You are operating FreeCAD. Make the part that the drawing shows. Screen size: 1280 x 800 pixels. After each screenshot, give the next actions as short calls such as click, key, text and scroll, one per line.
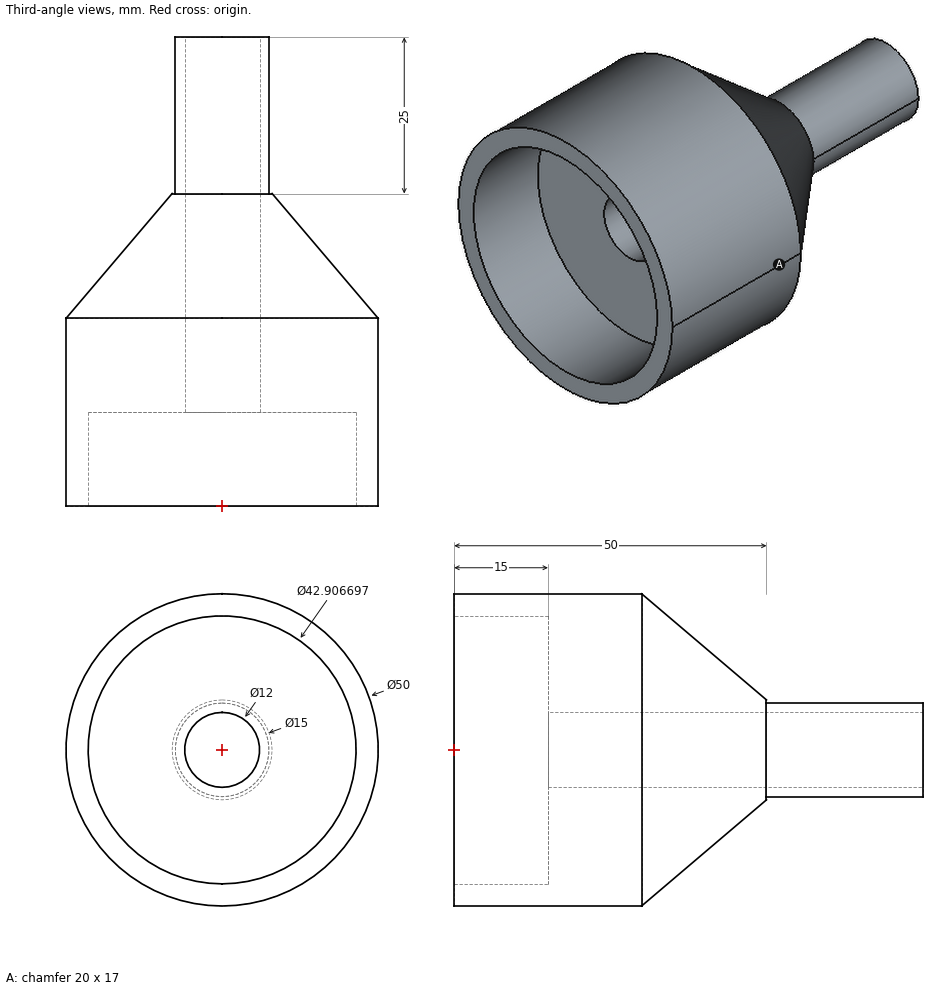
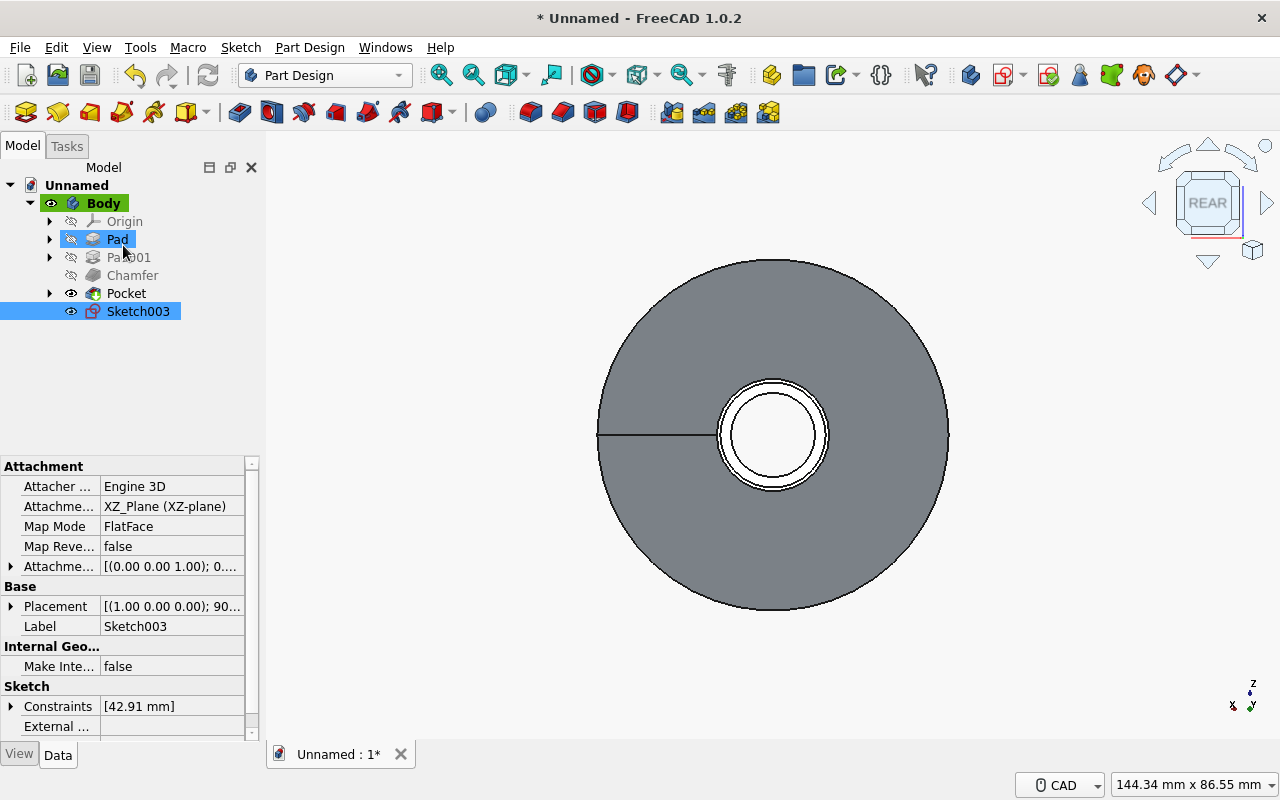
click(240, 112)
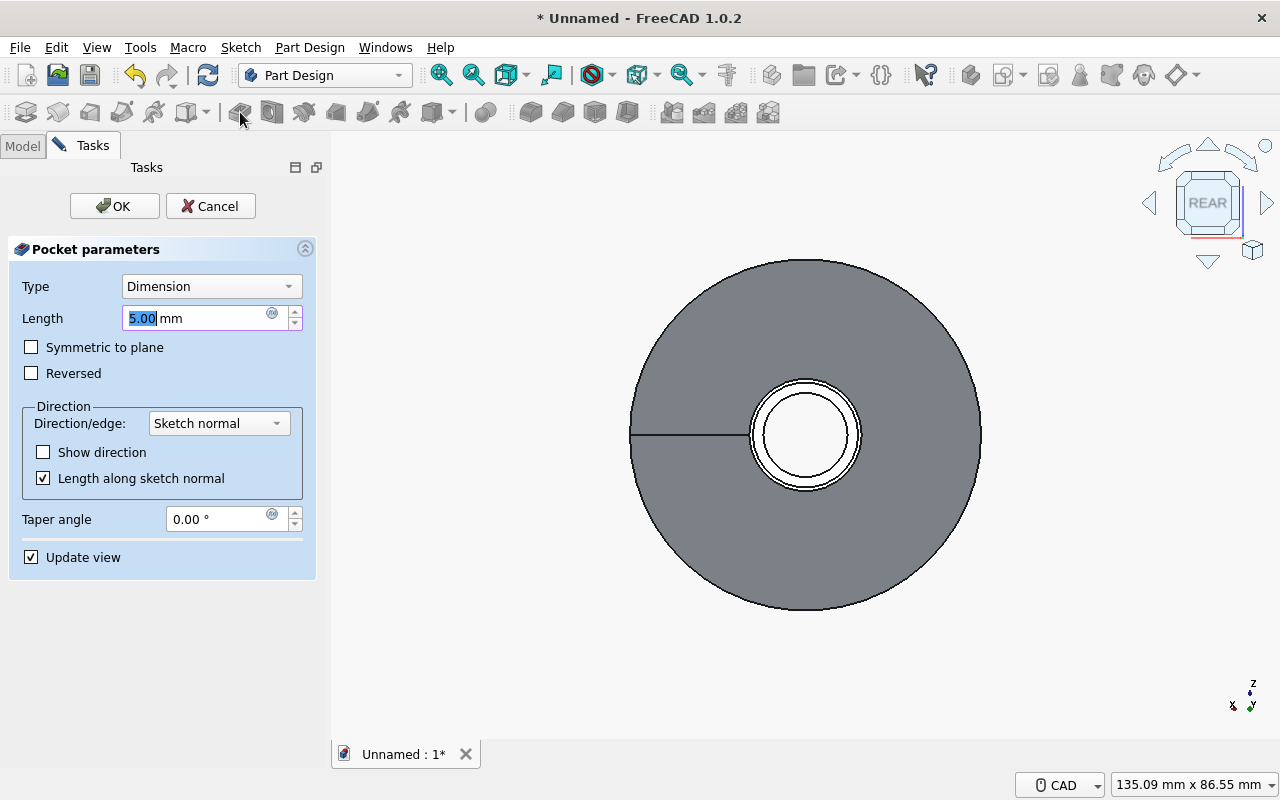
text(15)
key(Tab)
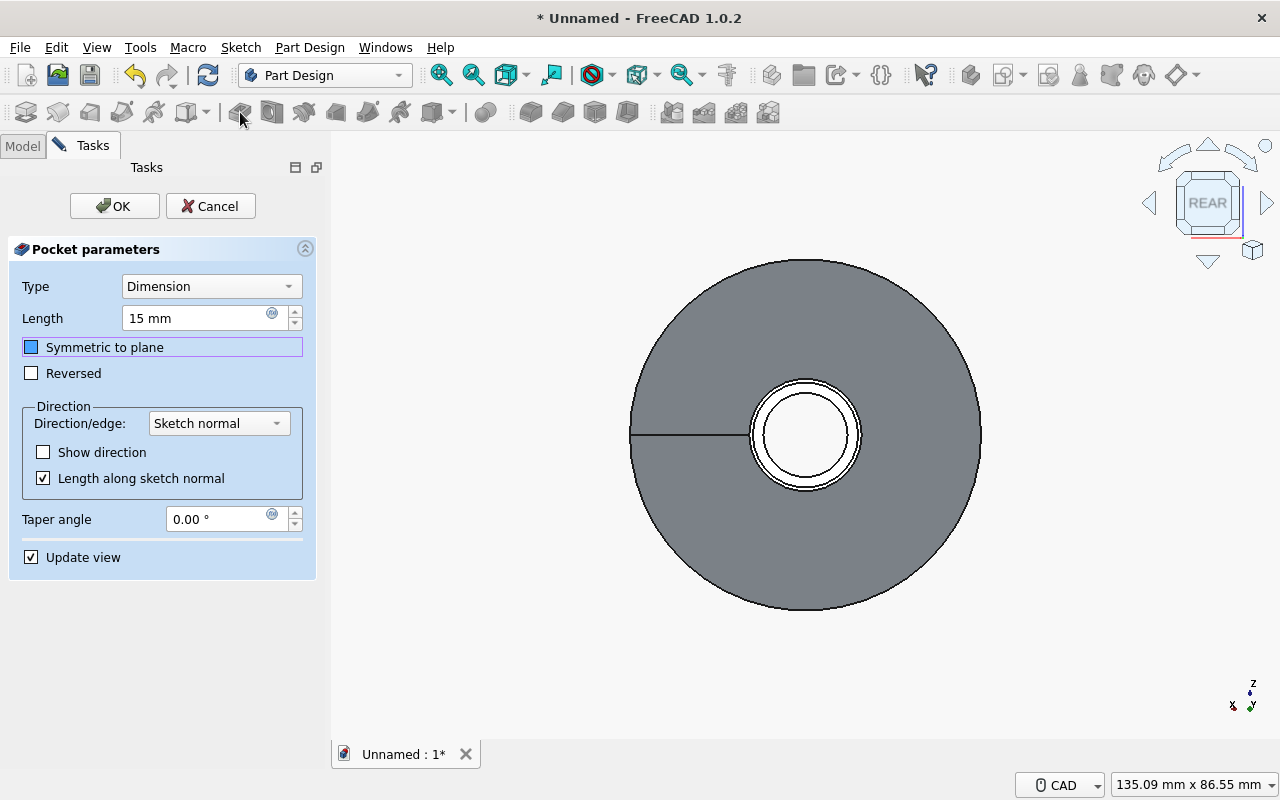
click(115, 206)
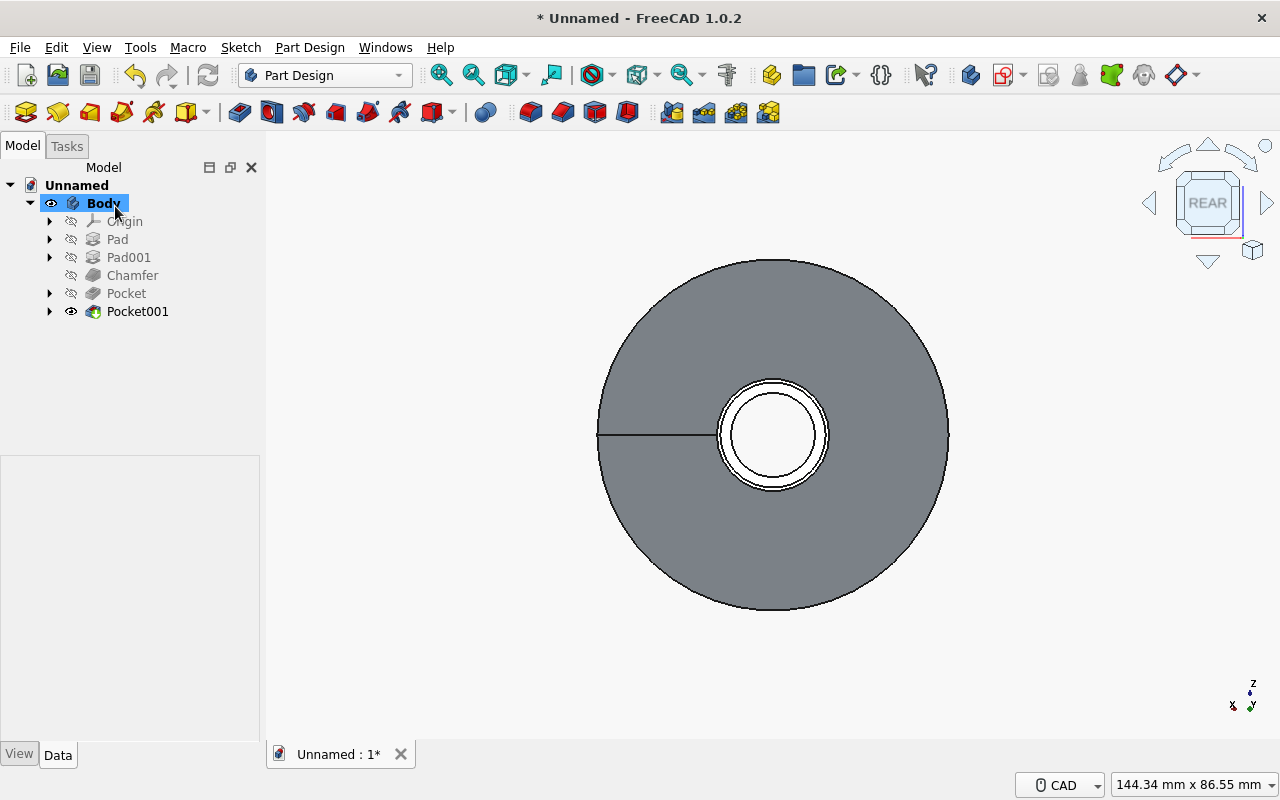
key(0)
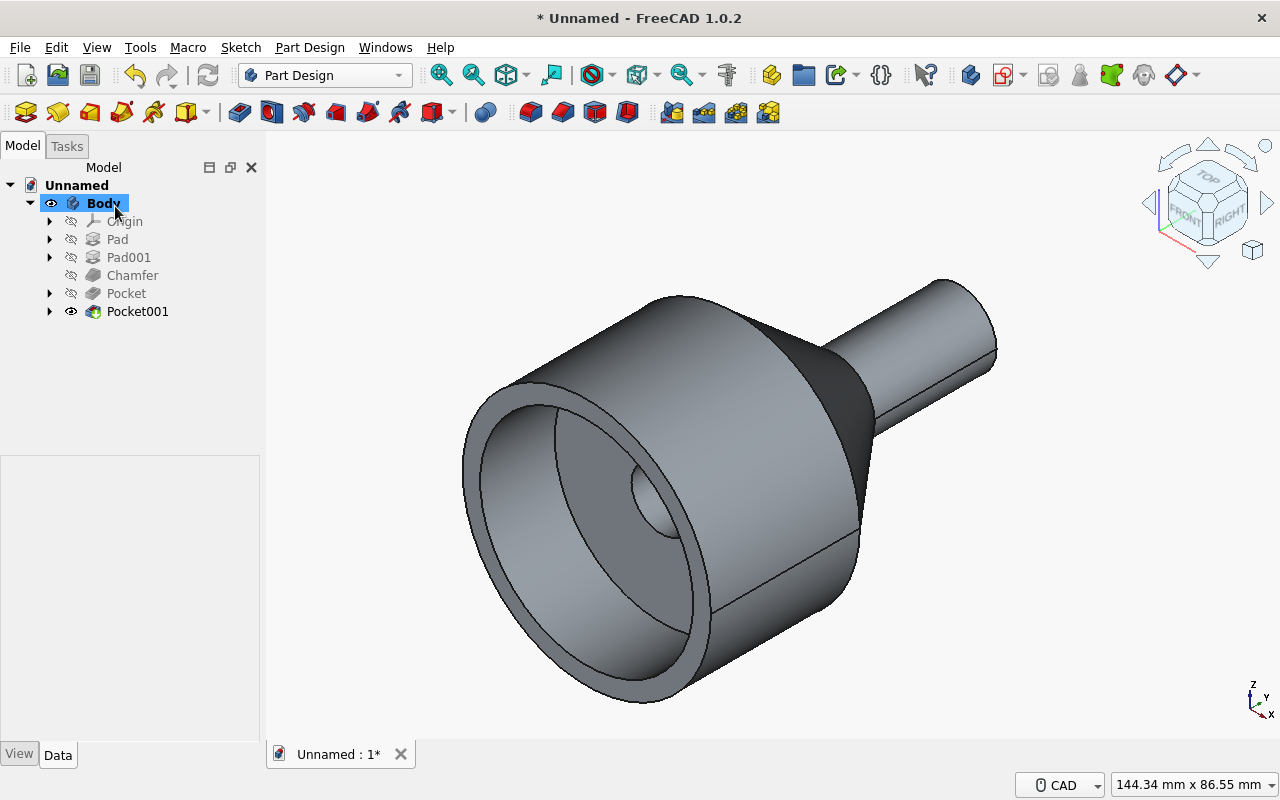
click(442, 76)